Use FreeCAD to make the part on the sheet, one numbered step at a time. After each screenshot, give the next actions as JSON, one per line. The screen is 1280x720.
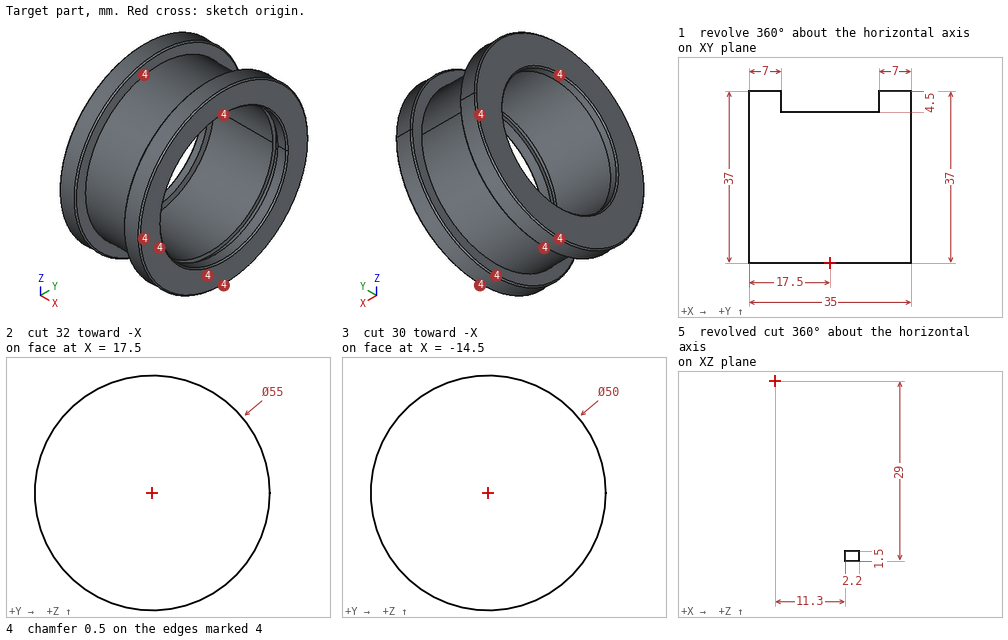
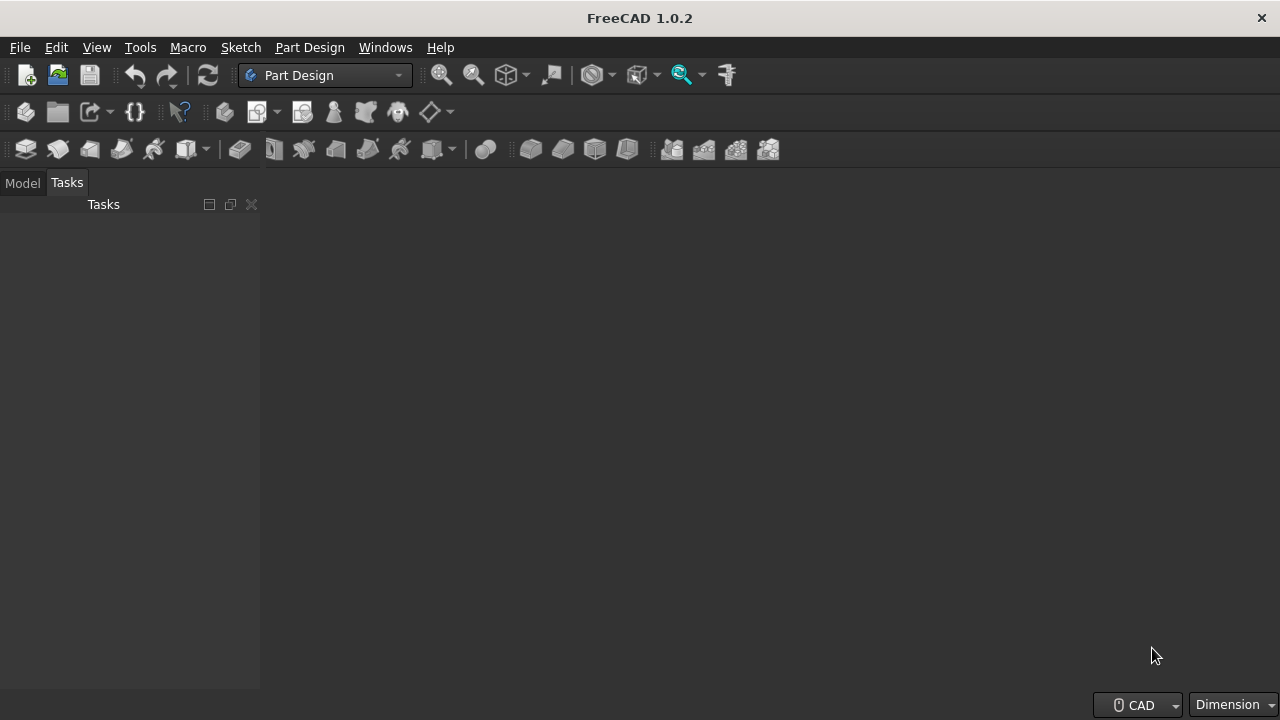
{"action": "left_click", "coordinate": [212, 76]}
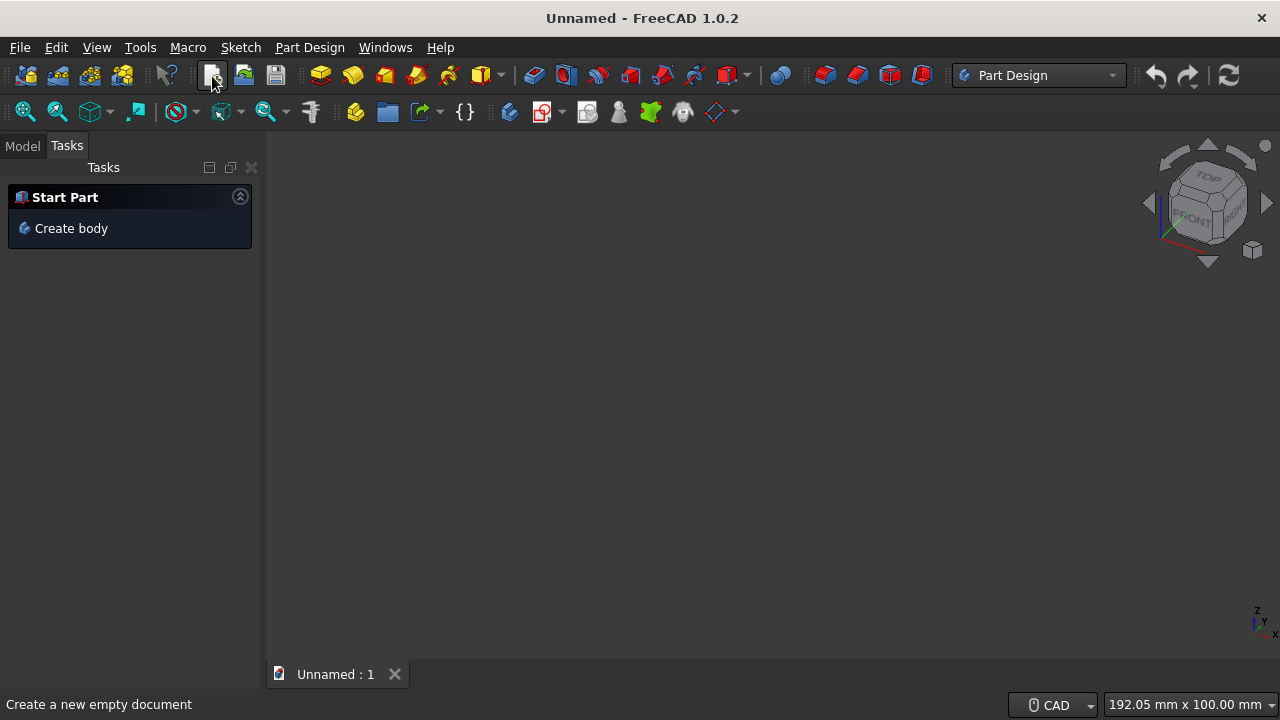
{"action": "left_click", "coordinate": [542, 112]}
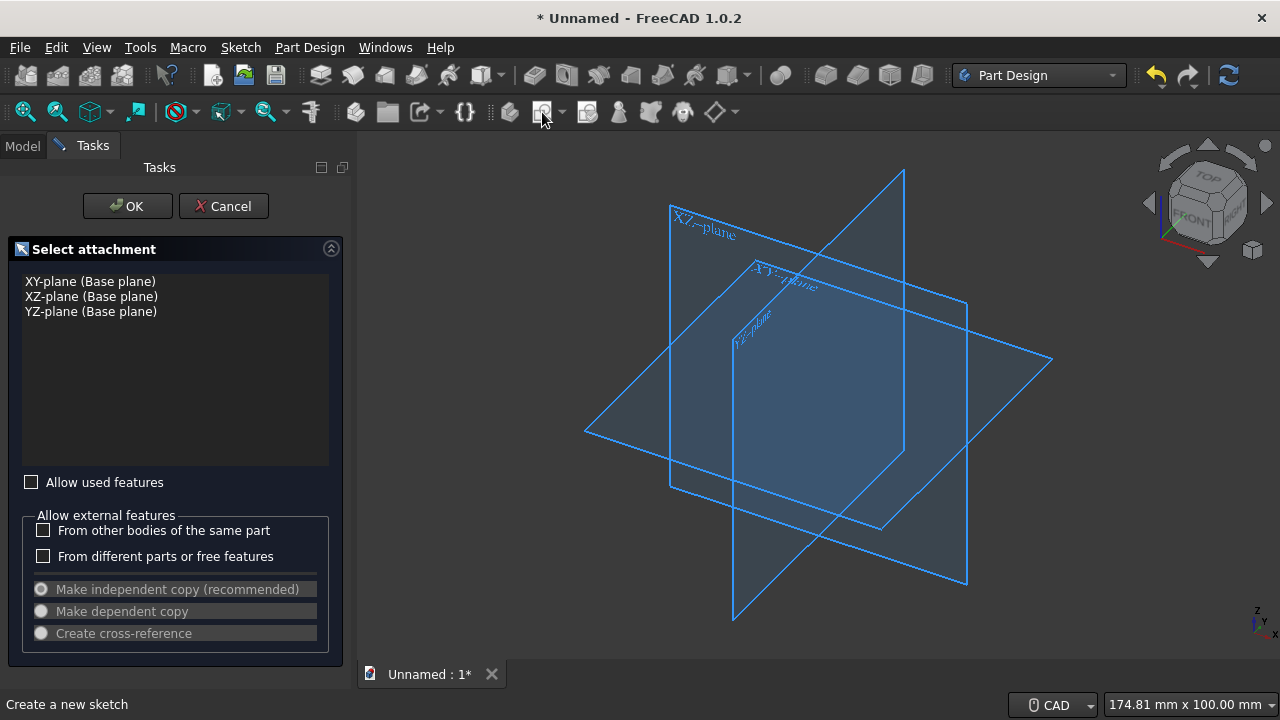
{"action": "left_click", "coordinate": [82, 282]}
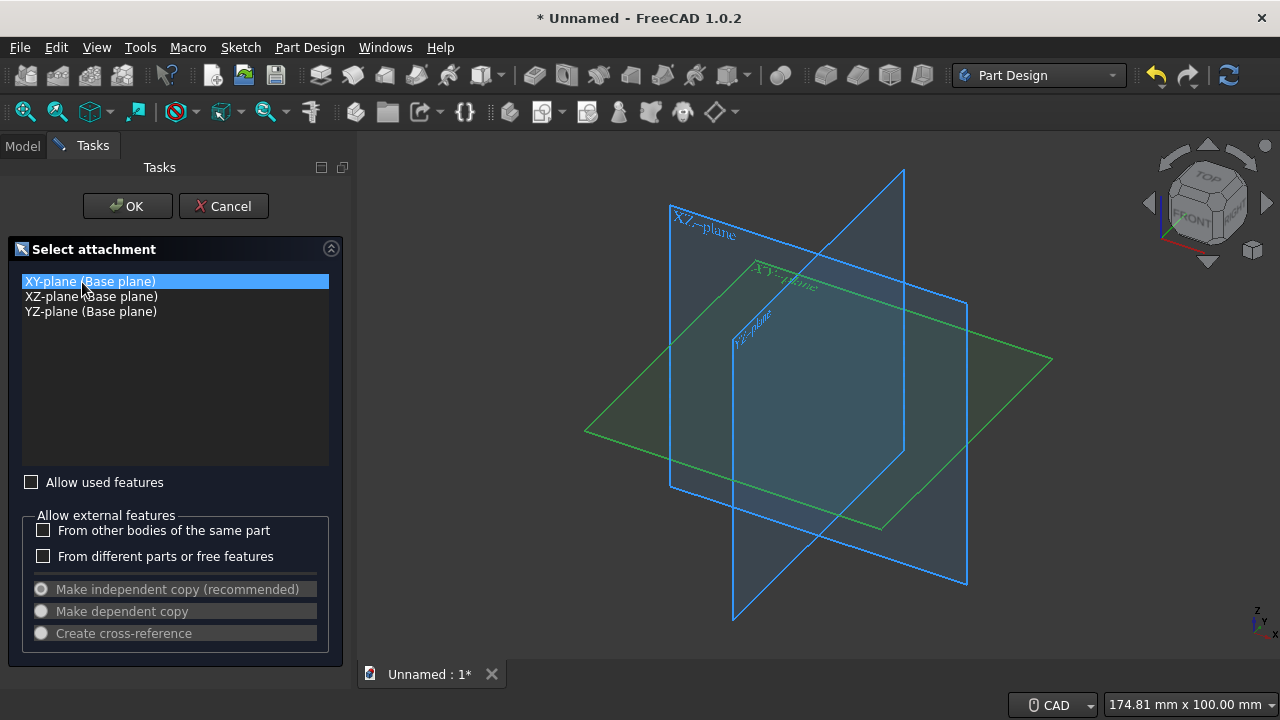
{"action": "left_click", "coordinate": [128, 206]}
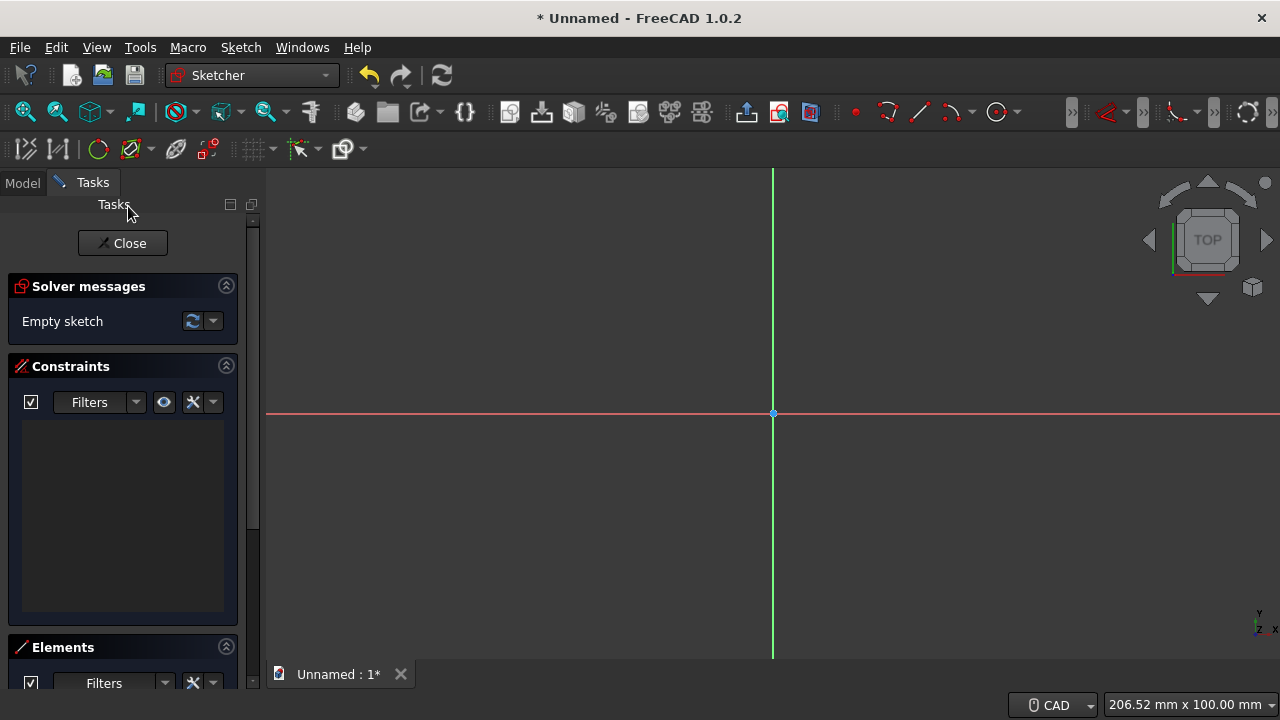
{"action": "scroll", "coordinate": [856, 212], "scroll_direction": "up", "scroll_amount": 3}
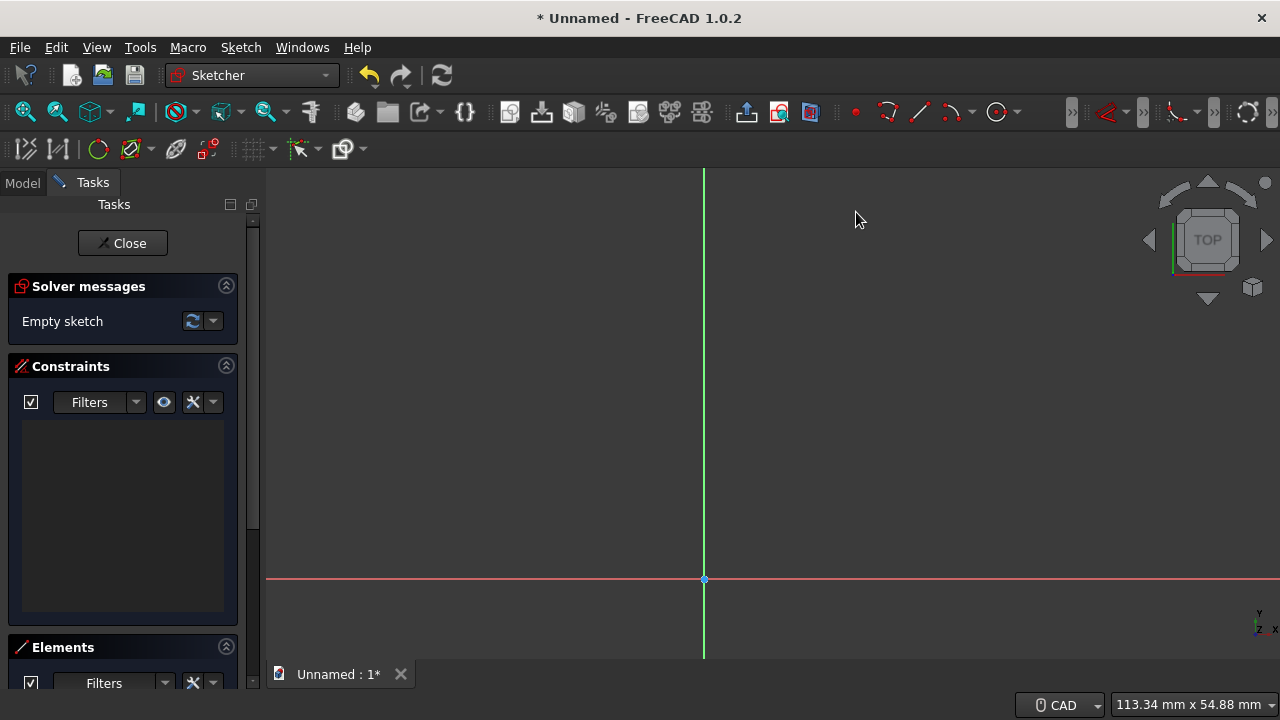
{"action": "left_click", "coordinate": [888, 112]}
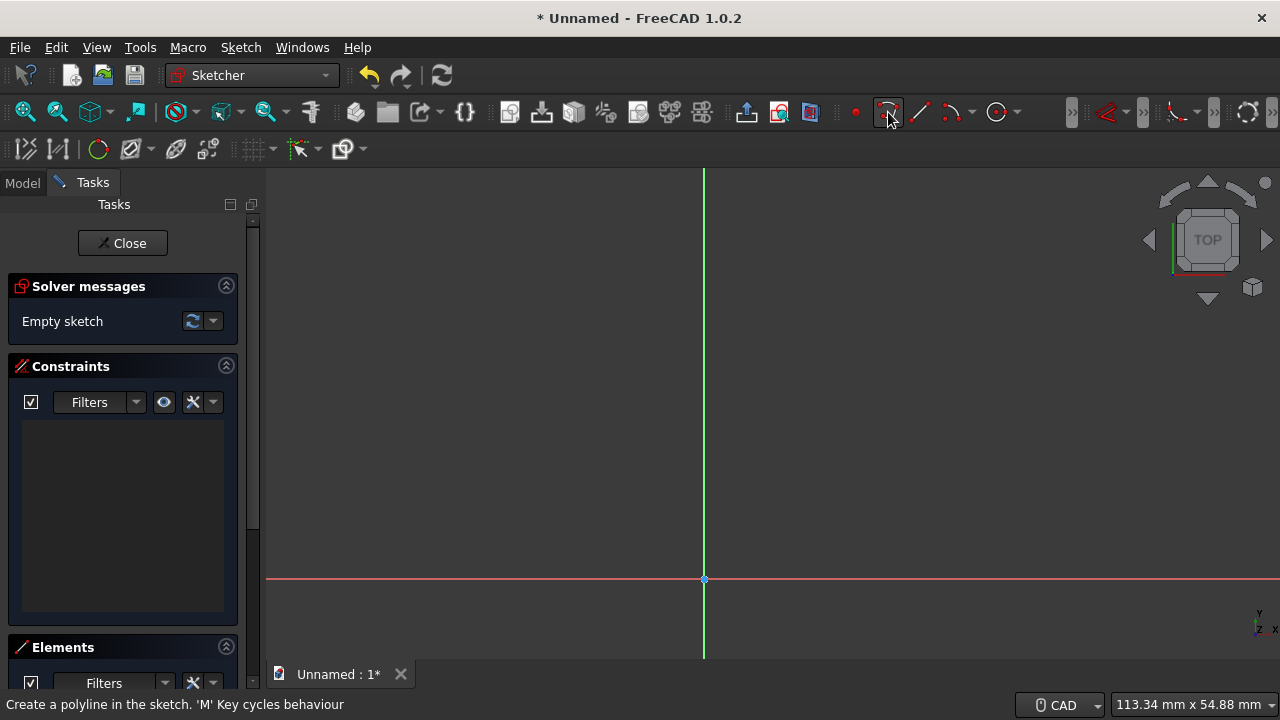
{"action": "left_click", "coordinate": [548, 579]}
{"action": "left_click", "coordinate": [861, 570]}
{"action": "left_click", "coordinate": [861, 248]}
{"action": "left_click", "coordinate": [798, 248]}
{"action": "left_click", "coordinate": [798, 288]}
{"action": "left_click", "coordinate": [610, 288]}
{"action": "left_click", "coordinate": [610, 248]}
{"action": "left_click", "coordinate": [548, 248]}
{"action": "left_click", "coordinate": [548, 579]}
{"action": "key", "text": "Escape"}
{"action": "key", "text": "Escape"}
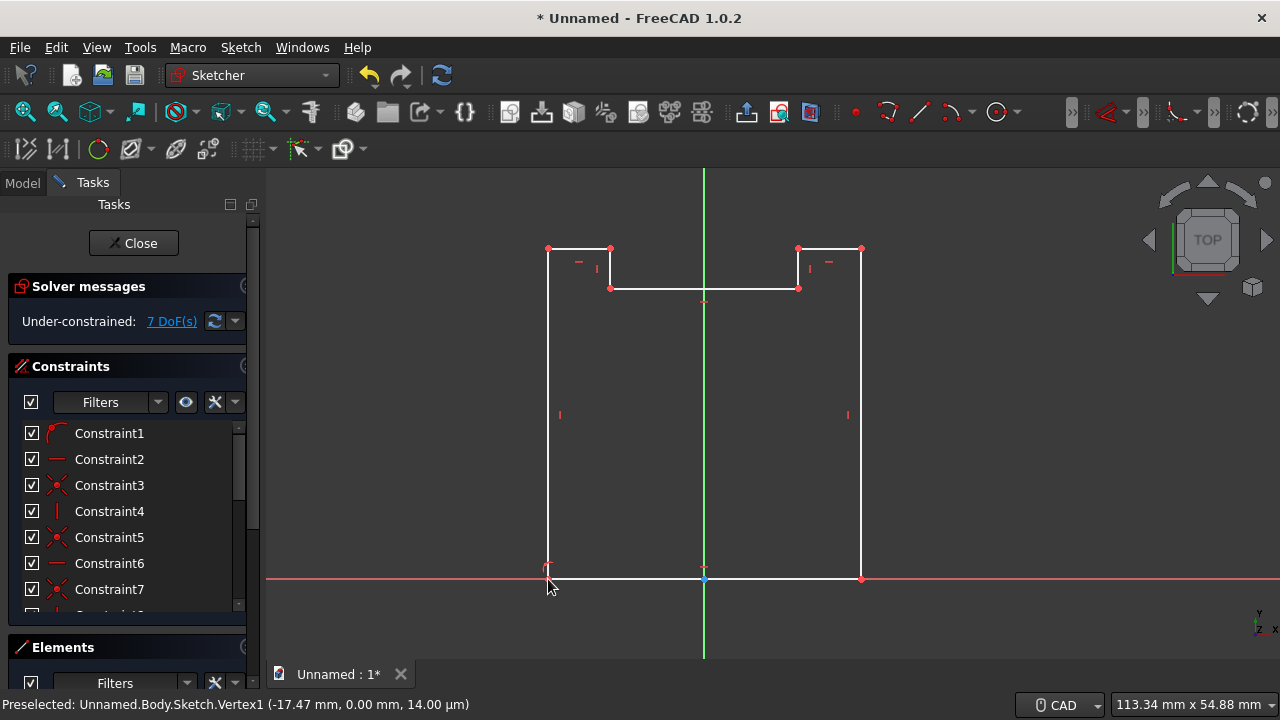
{"action": "left_click", "coordinate": [1106, 112]}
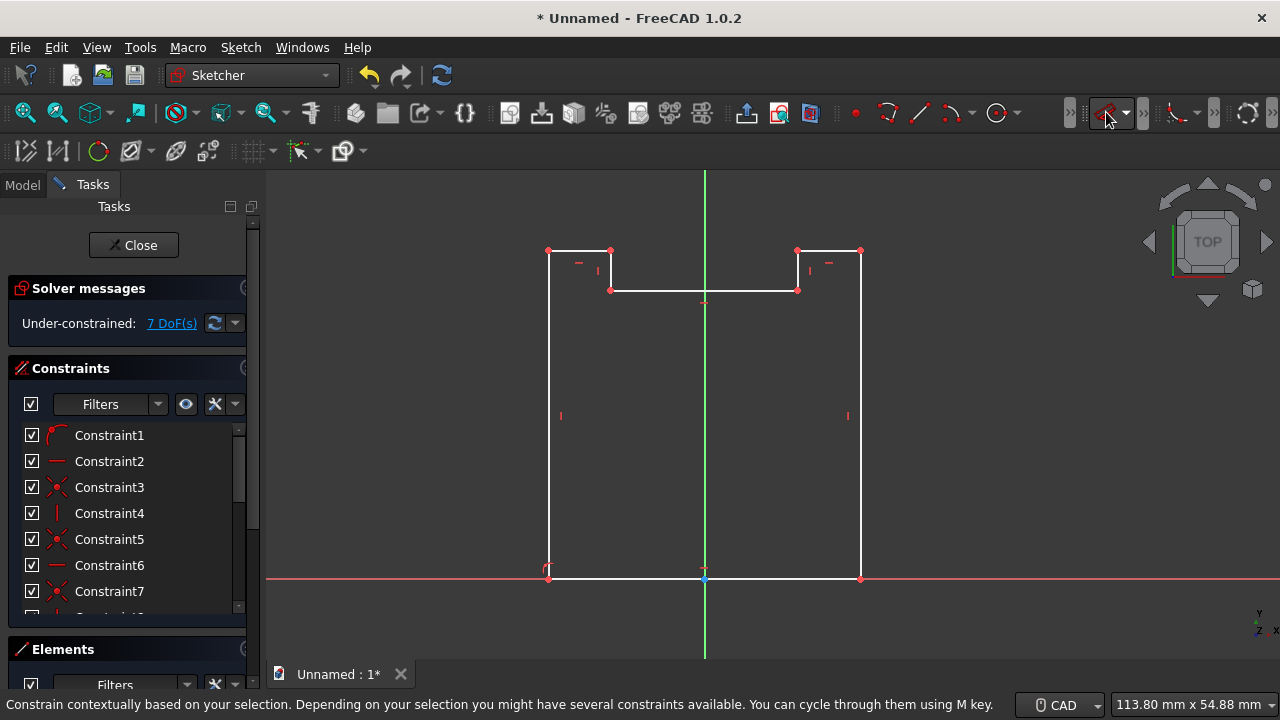
{"action": "left_click", "coordinate": [842, 251]}
{"action": "left_click", "coordinate": [829, 217]}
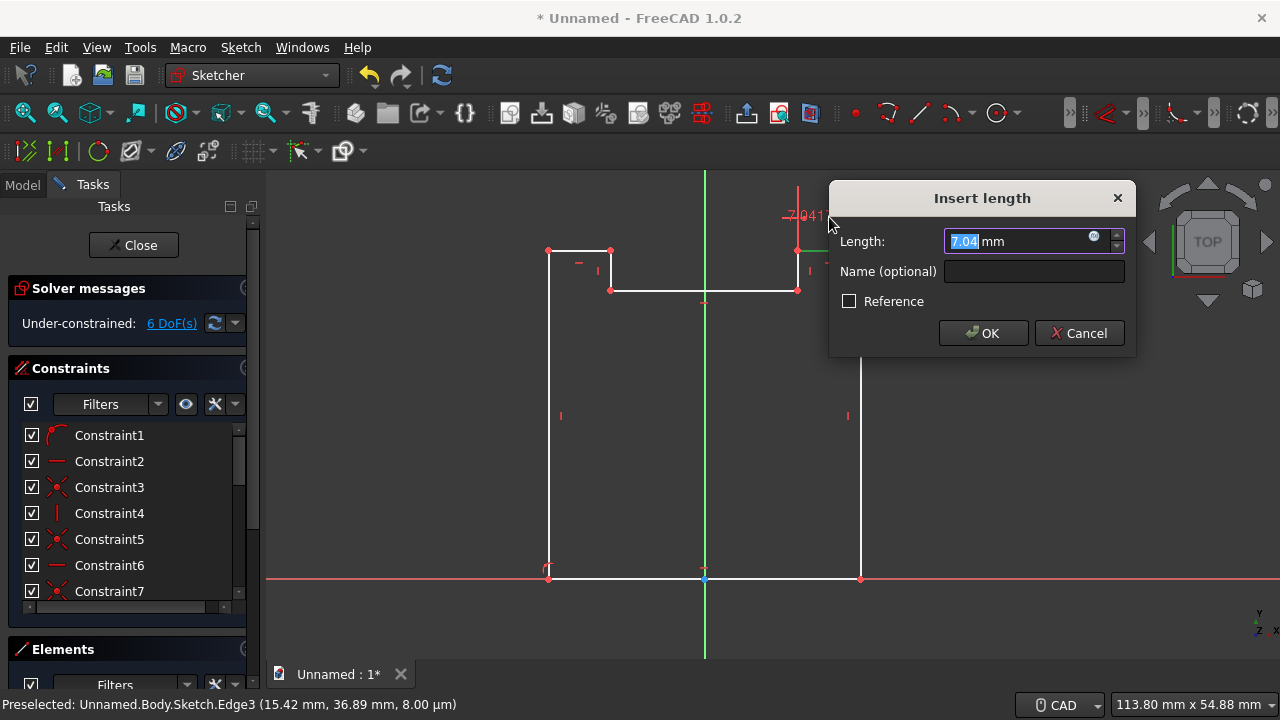
{"action": "type", "text": "7"}
{"action": "key", "text": "Return"}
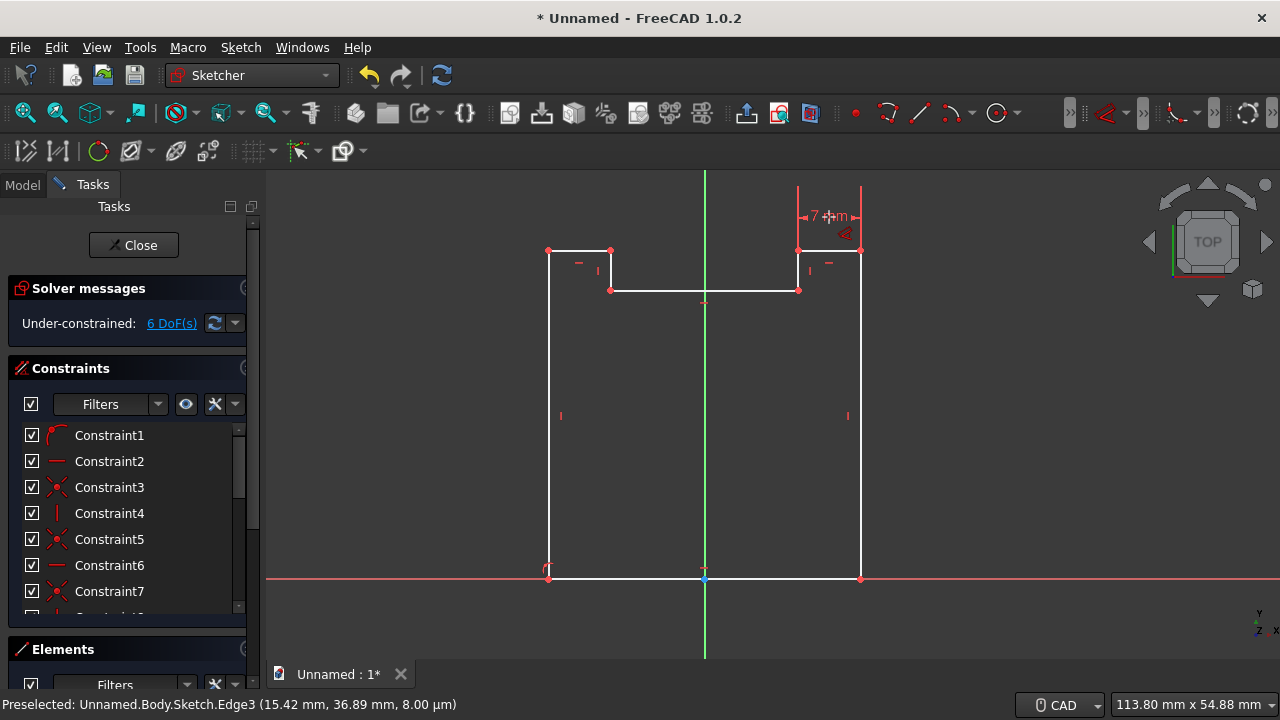
{"action": "left_click", "coordinate": [592, 251]}
{"action": "left_click", "coordinate": [580, 217]}